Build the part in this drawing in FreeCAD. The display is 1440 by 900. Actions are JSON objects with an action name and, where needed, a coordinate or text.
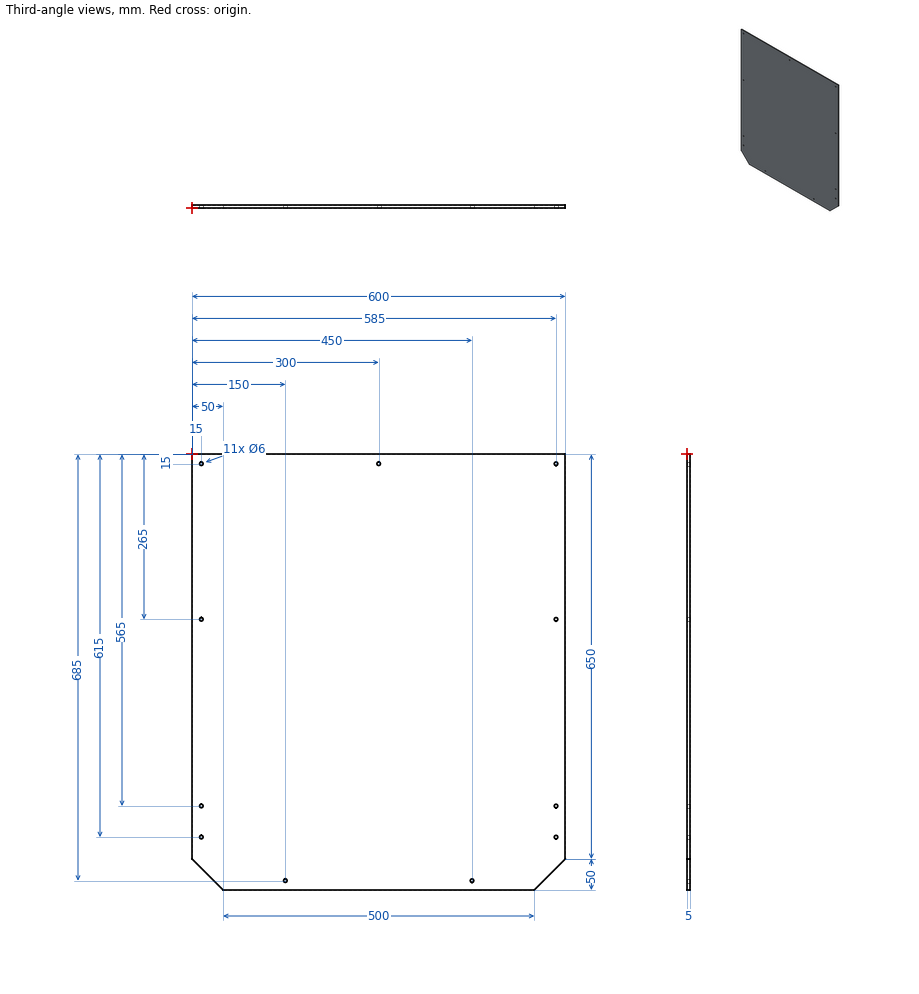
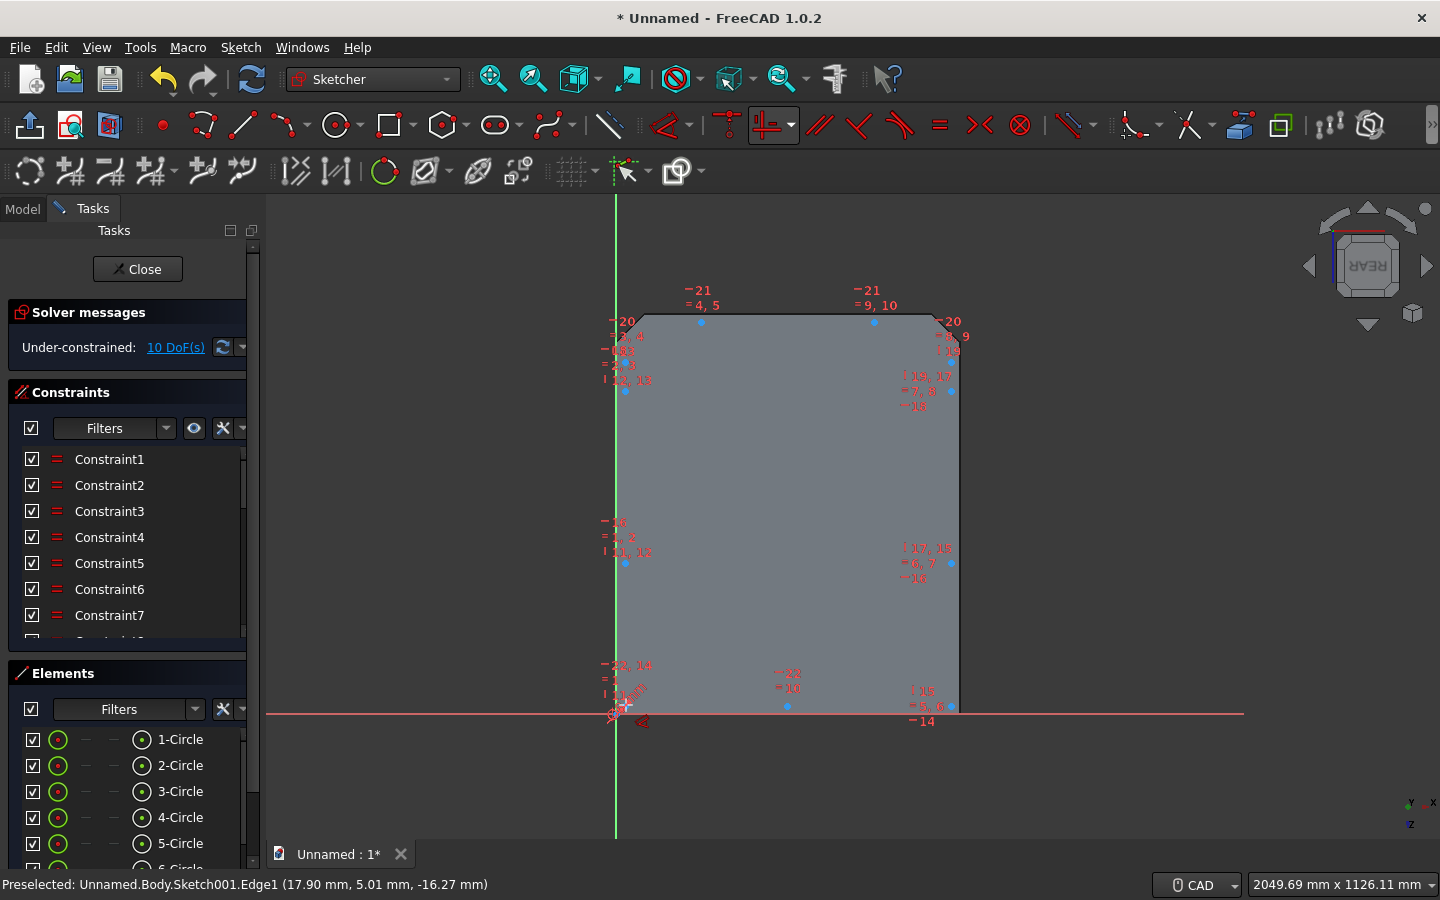
{"action": "scroll", "coordinate": [625, 706], "scroll_direction": "up", "scroll_amount": 8}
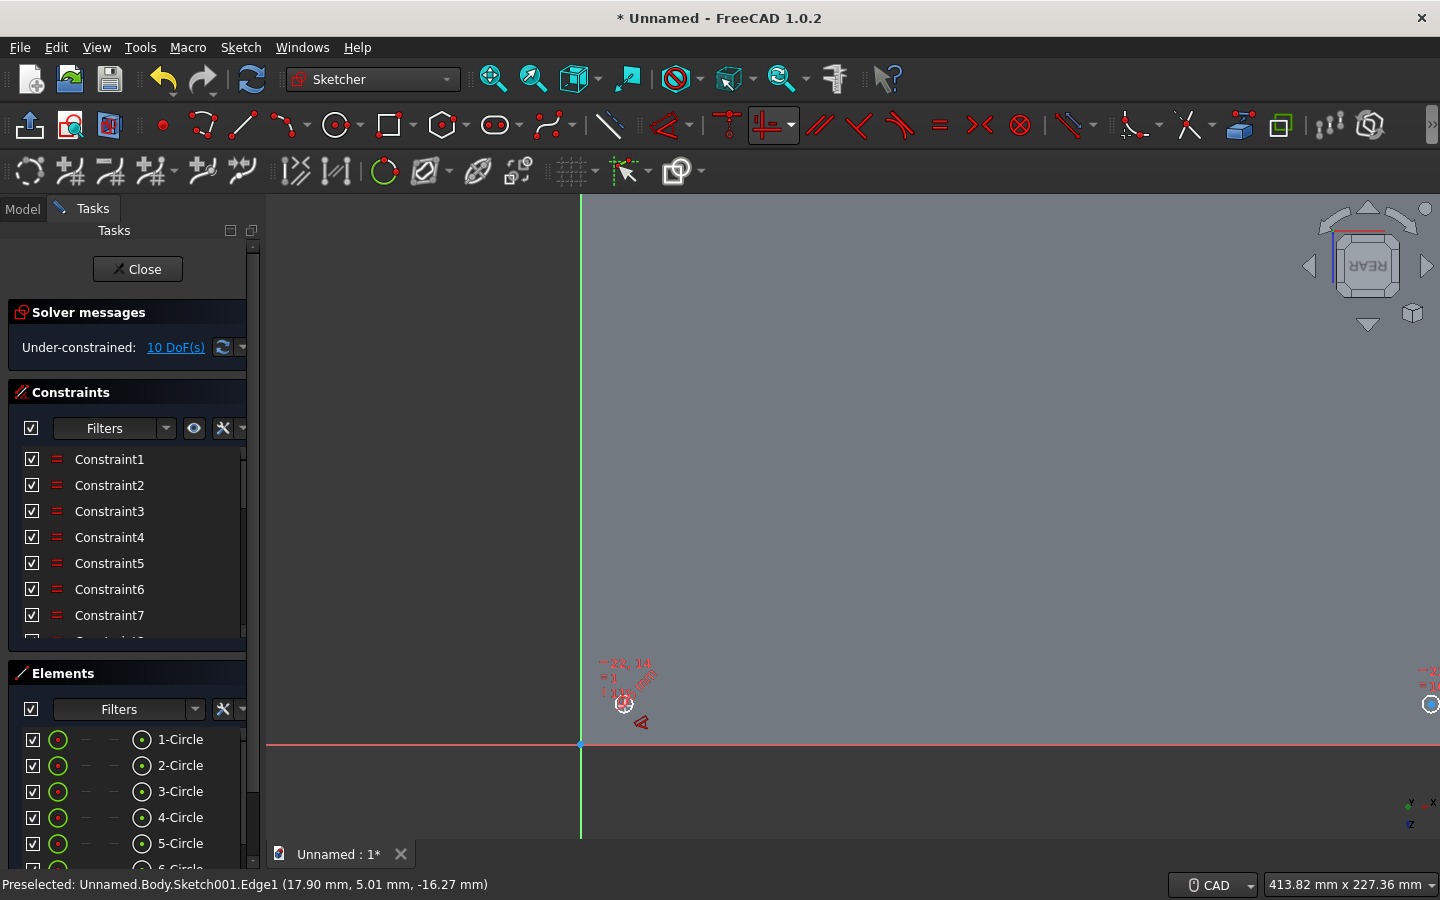
{"action": "left_click", "coordinate": [624, 704]}
{"action": "left_click", "coordinate": [602, 779]}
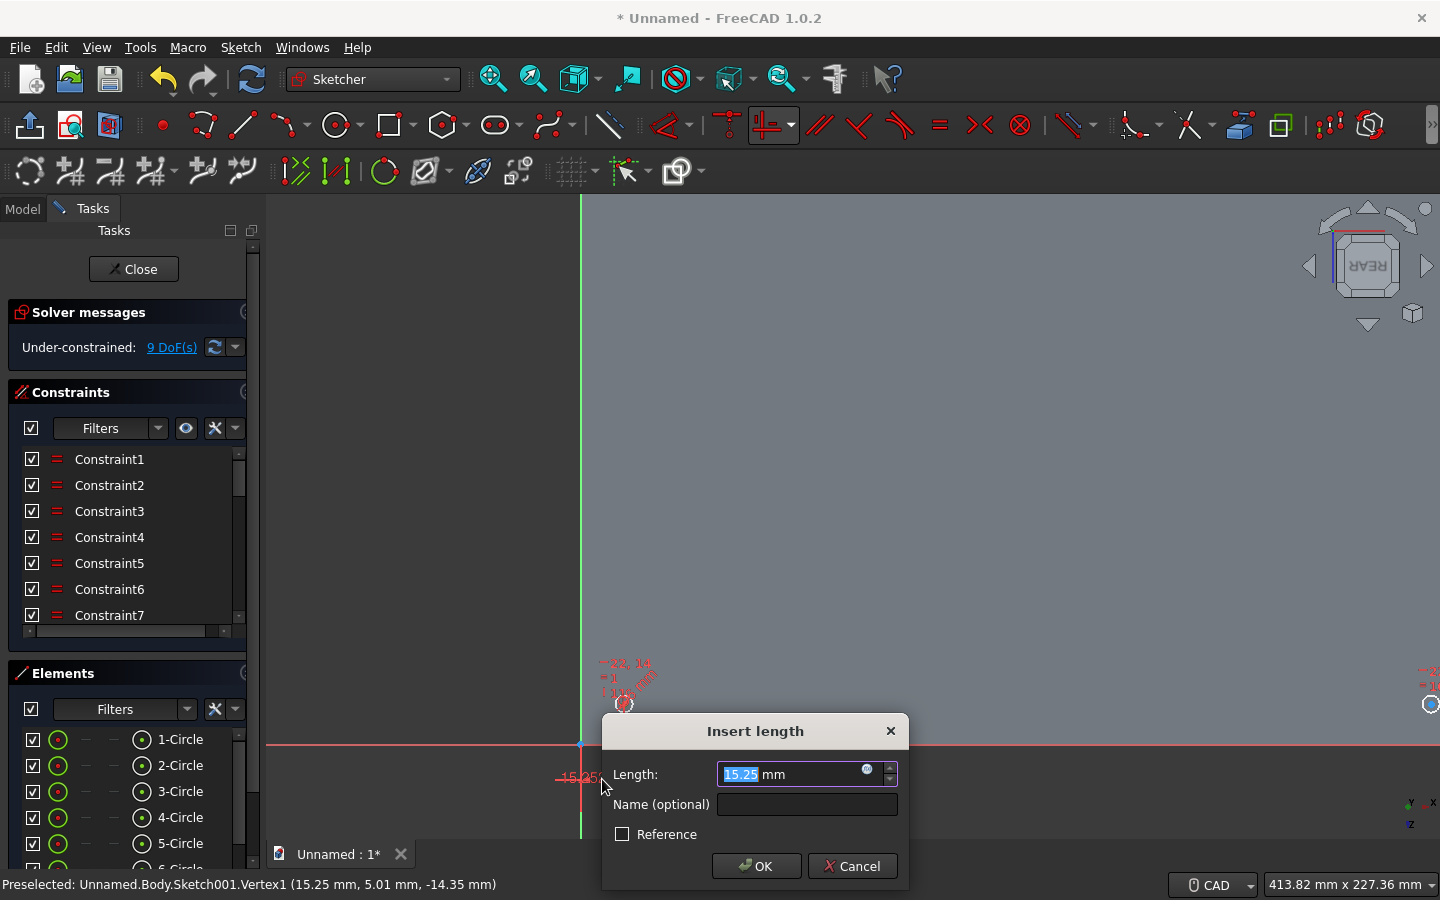
{"action": "type", "text": "15"}
{"action": "key", "text": "Return"}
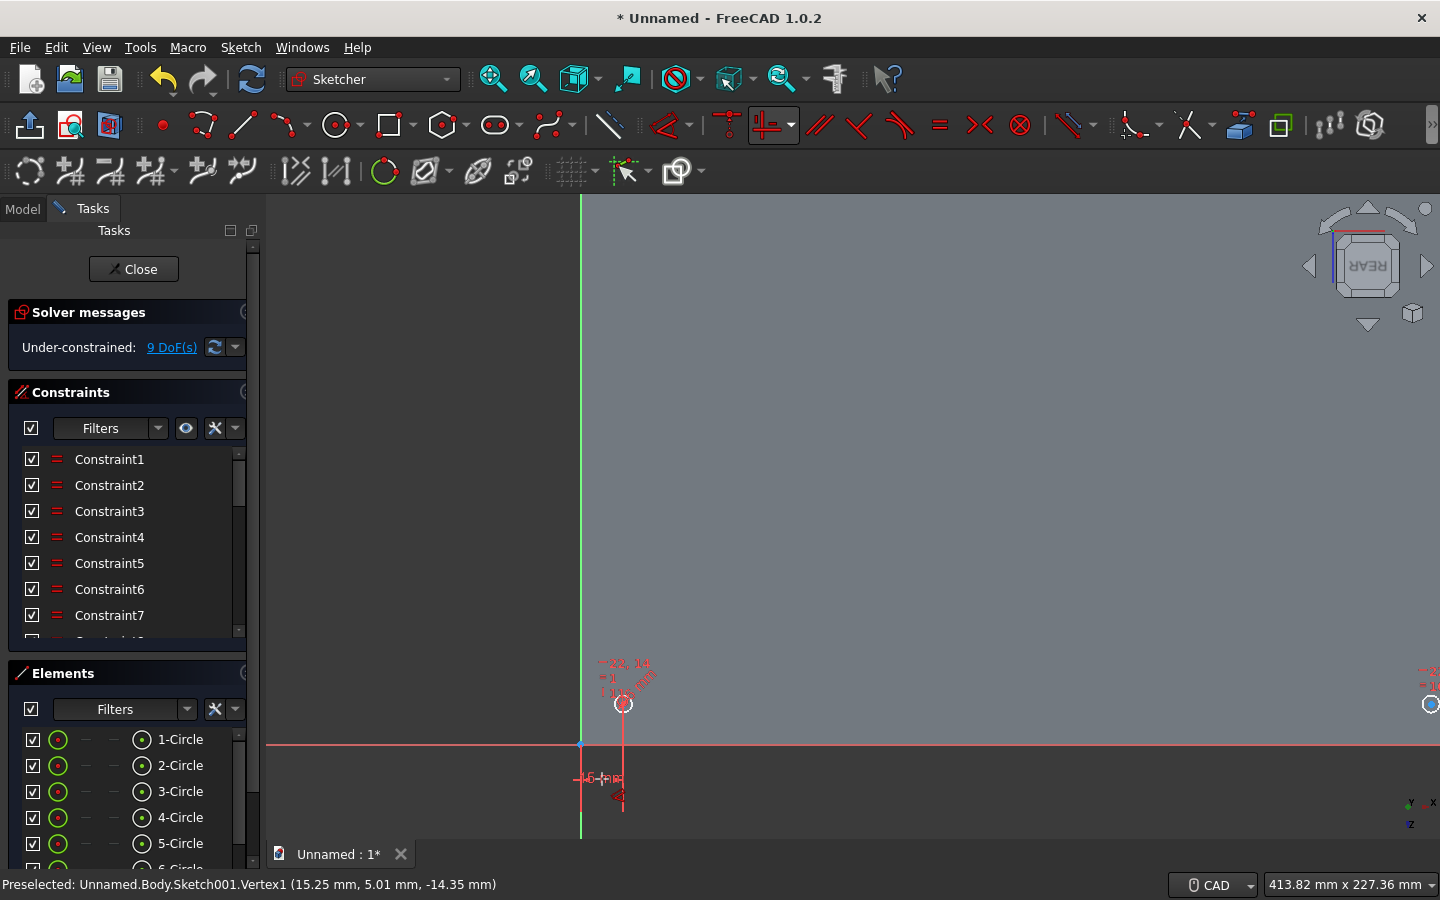
{"action": "left_click", "coordinate": [623, 704]}
{"action": "left_click", "coordinate": [547, 724]}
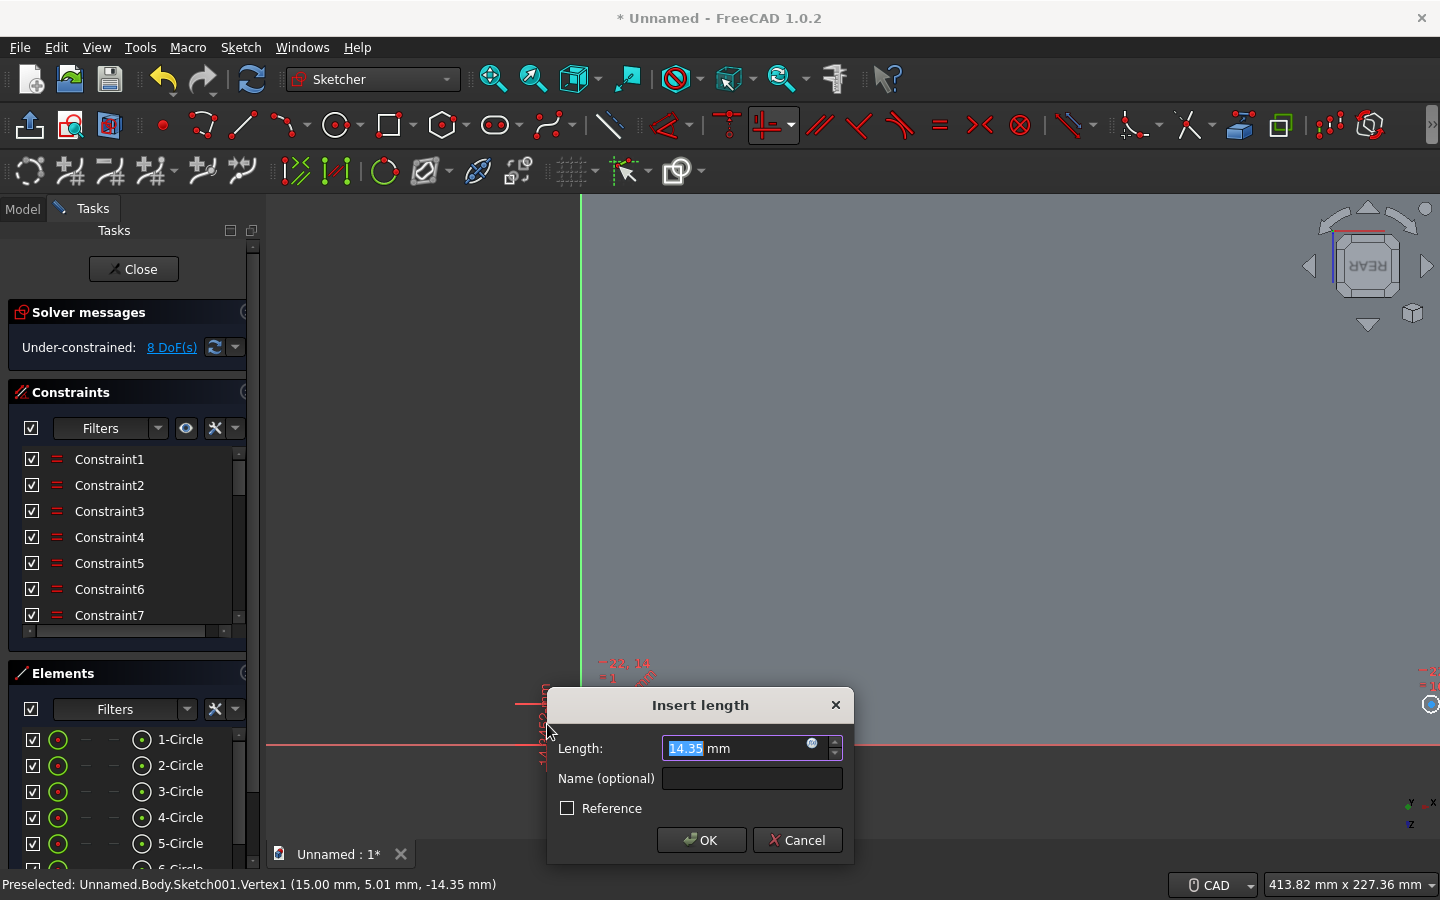
{"action": "type", "text": "15"}
{"action": "key", "text": "Return"}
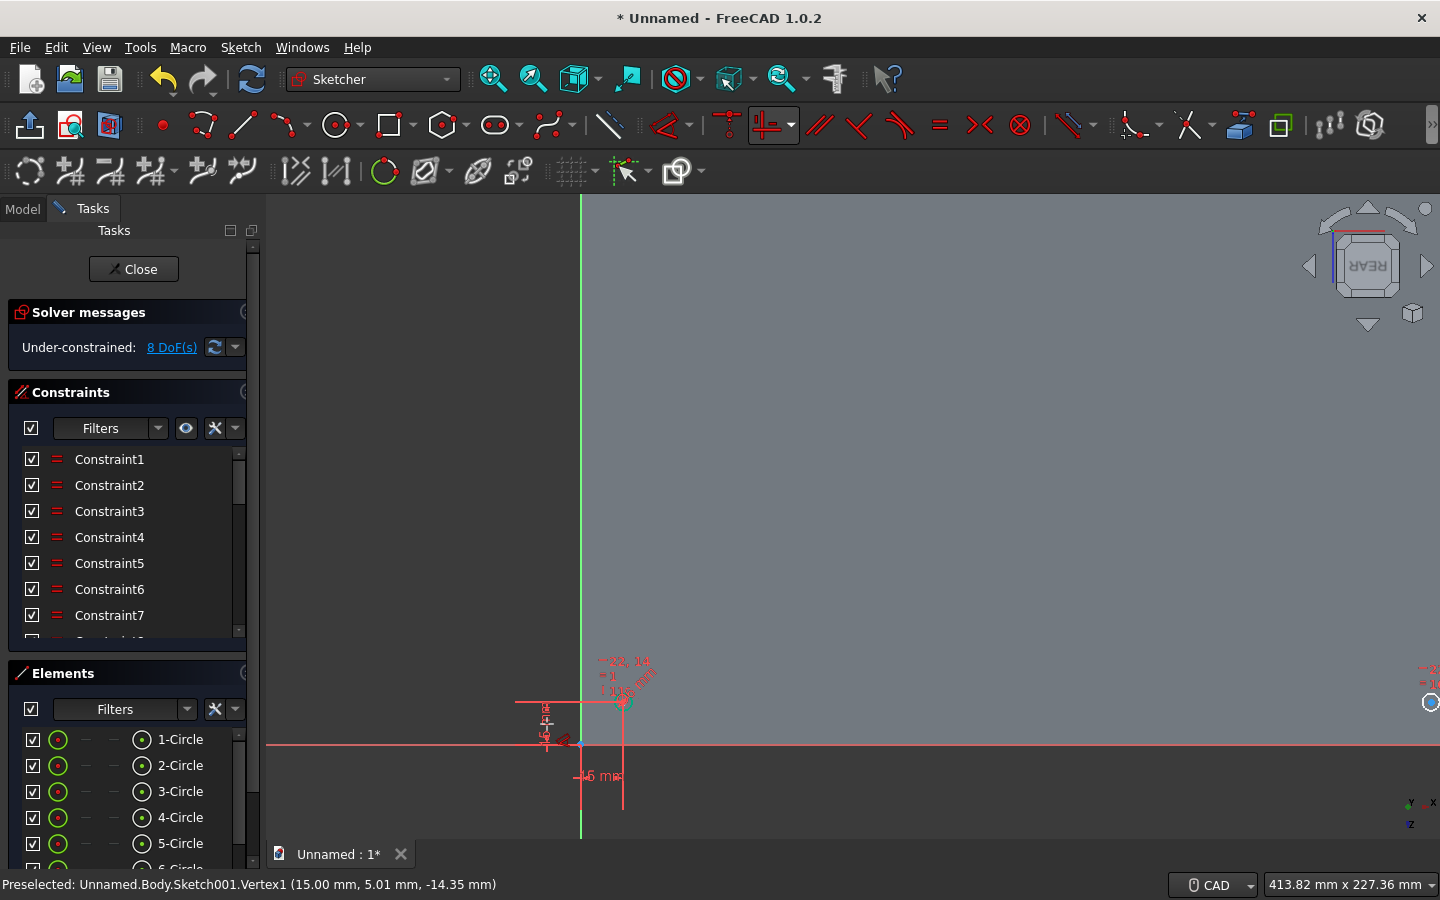
{"action": "scroll", "coordinate": [625, 706], "scroll_direction": "down", "scroll_amount": 8}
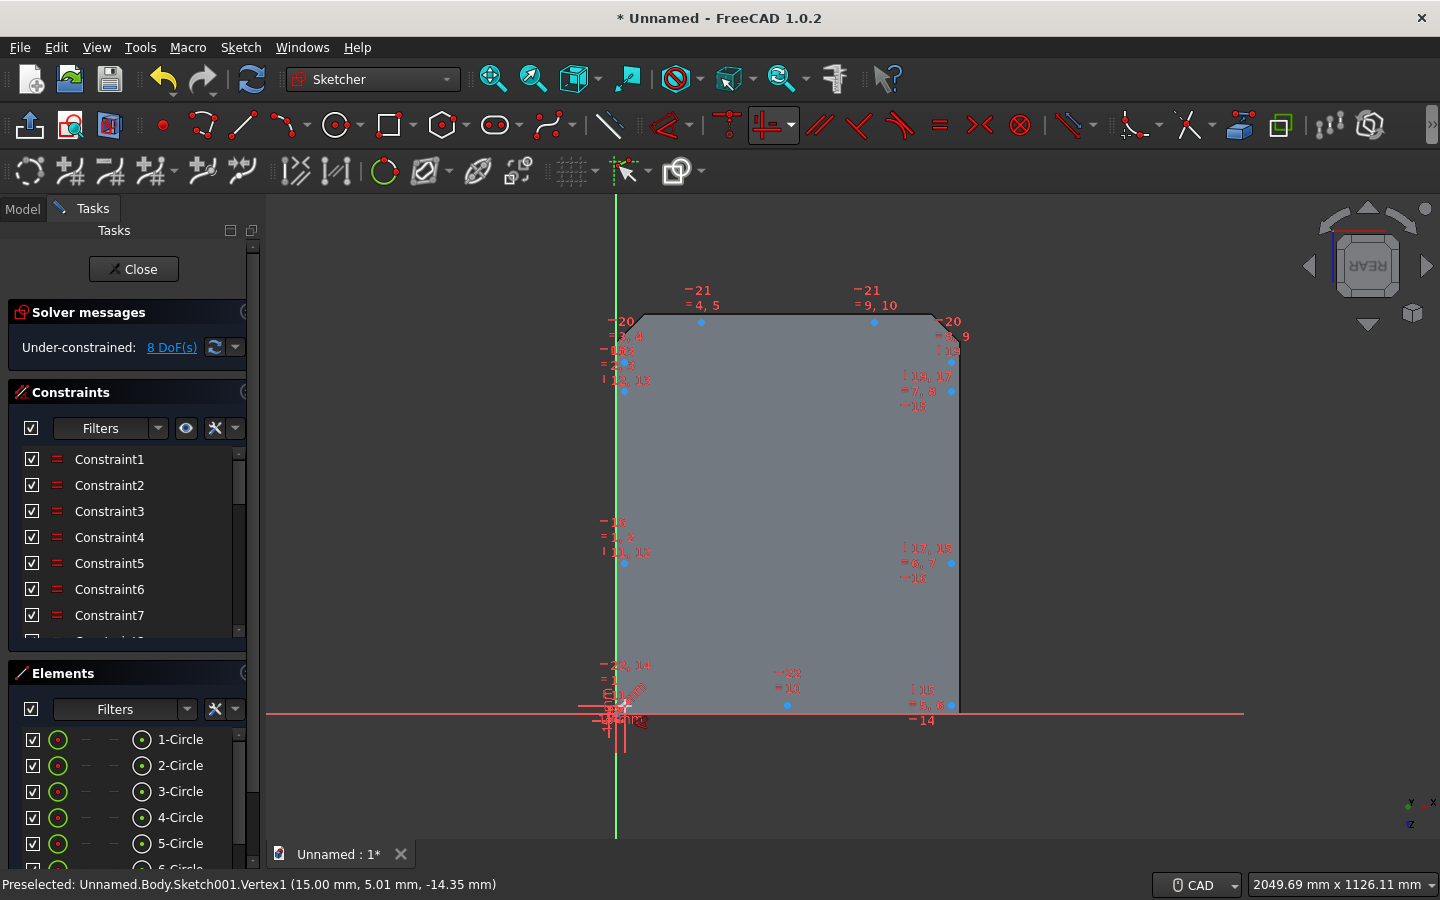
{"action": "left_click", "coordinate": [625, 563]}
{"action": "left_click", "coordinate": [582, 639]}